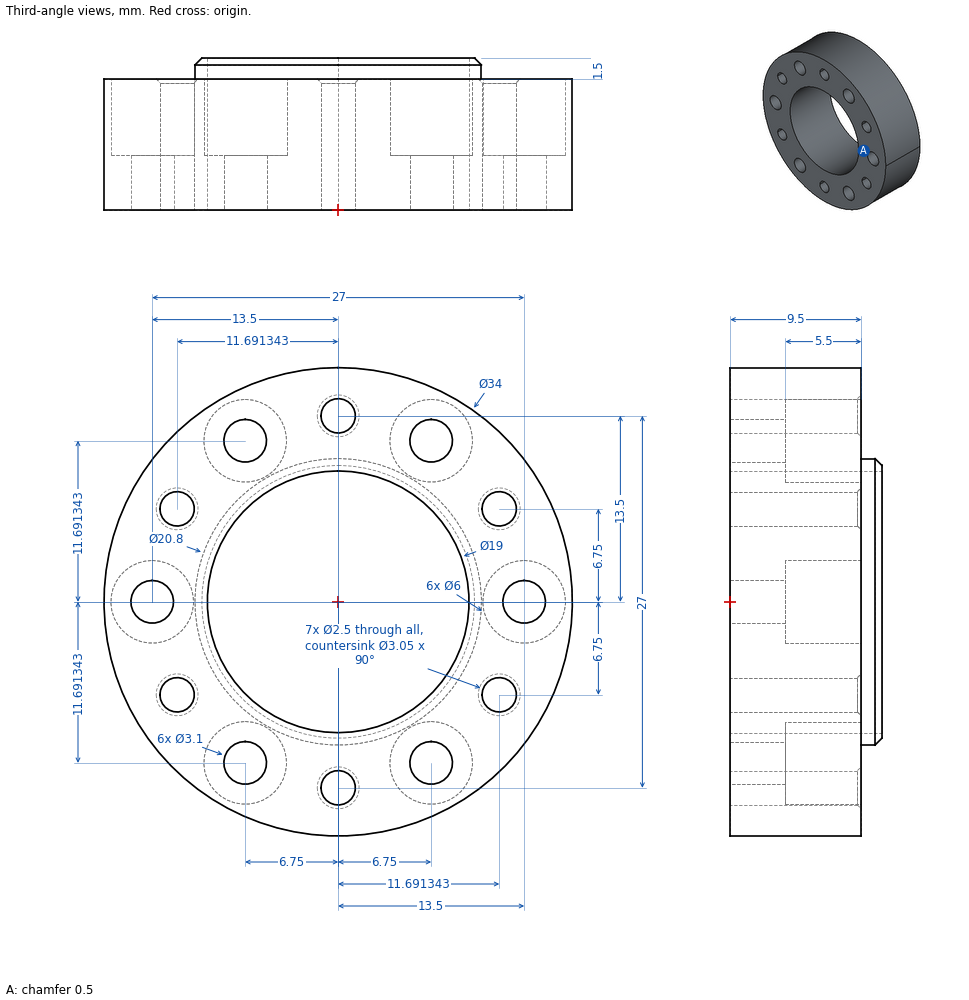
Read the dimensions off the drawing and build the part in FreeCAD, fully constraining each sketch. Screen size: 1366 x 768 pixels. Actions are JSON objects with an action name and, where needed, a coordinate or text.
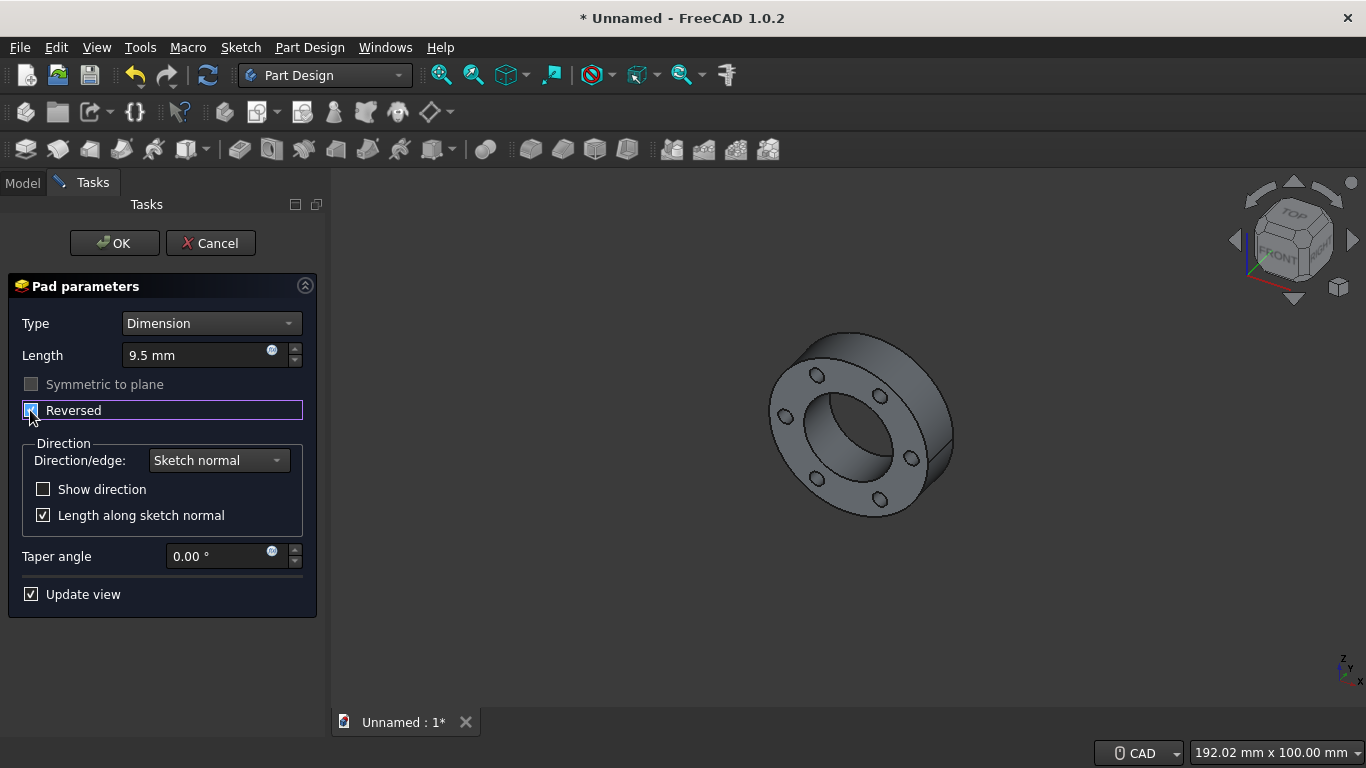
{"action": "left_click", "coordinate": [115, 243]}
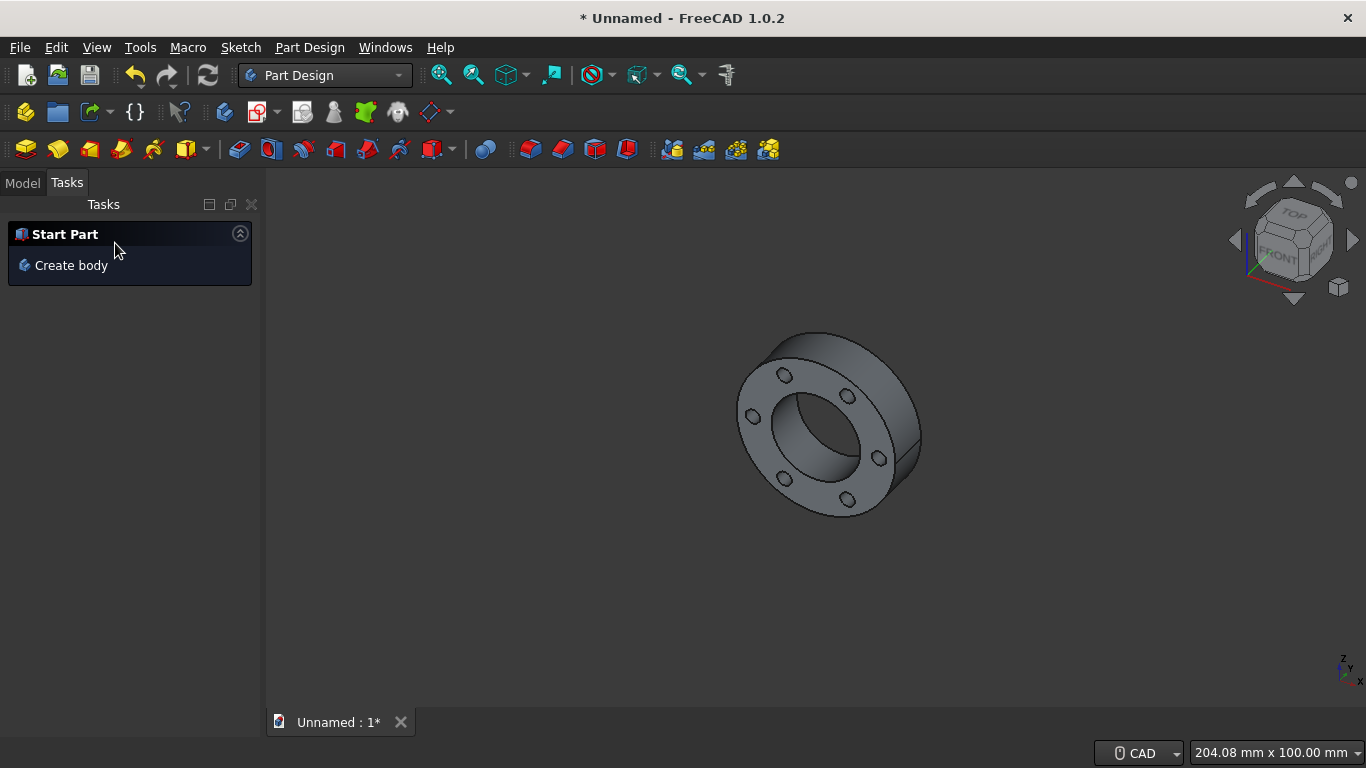
{"action": "left_click", "coordinate": [442, 76]}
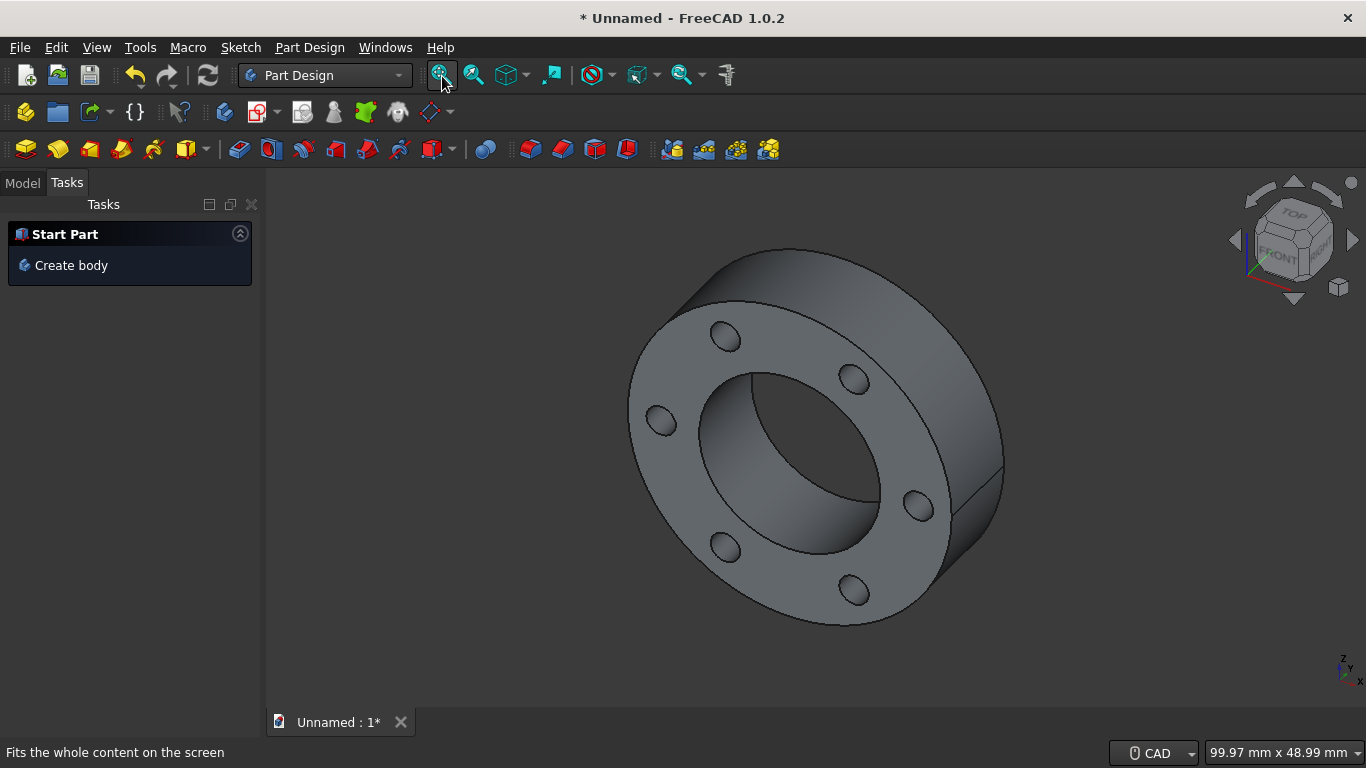
{"action": "key", "text": "4"}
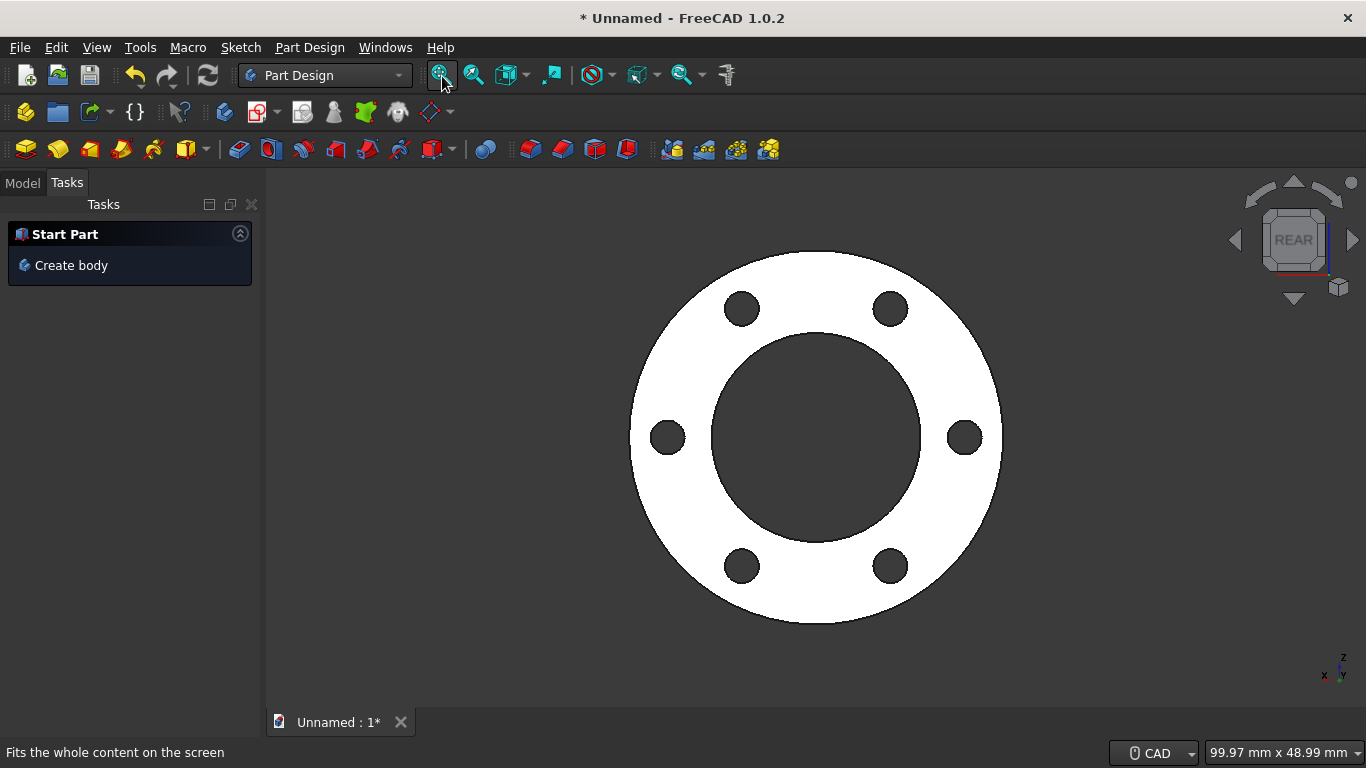
{"action": "left_click", "coordinate": [816, 597]}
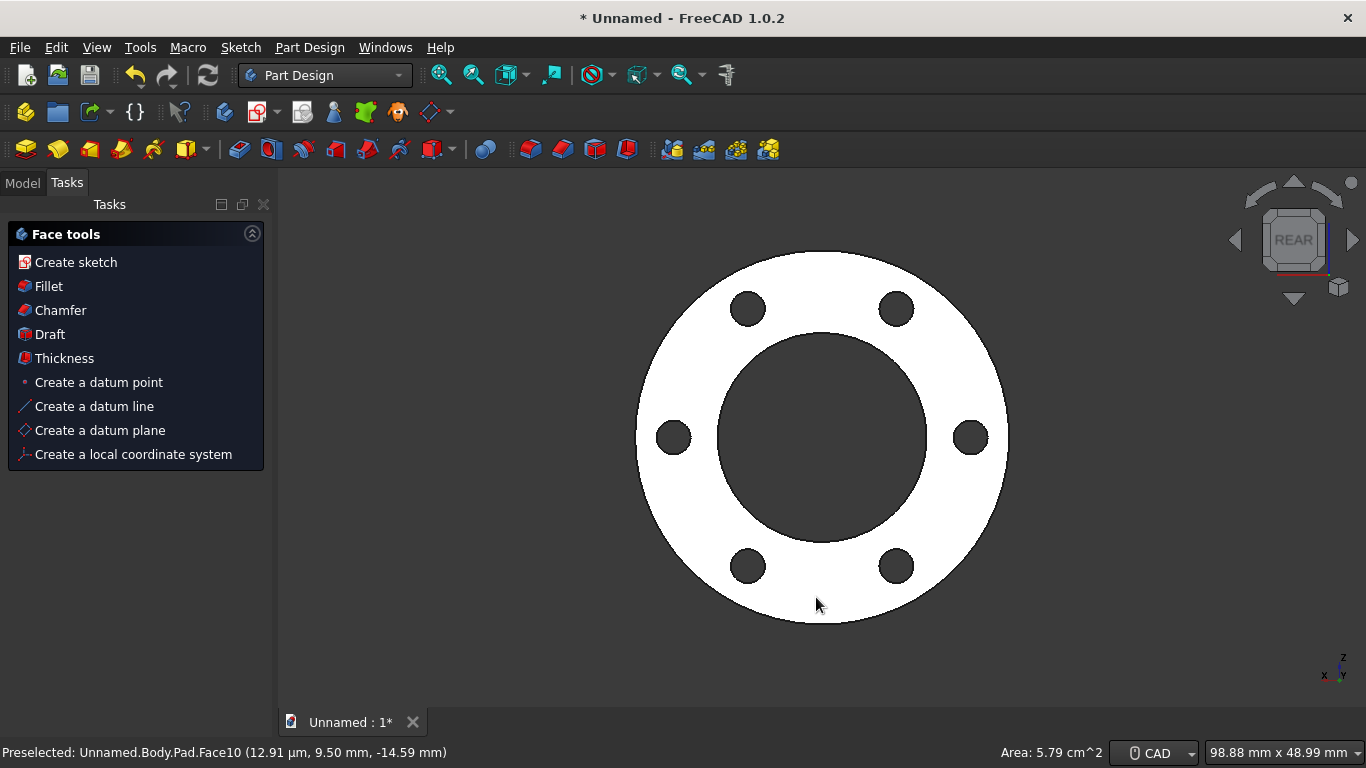
{"action": "left_click", "coordinate": [258, 112]}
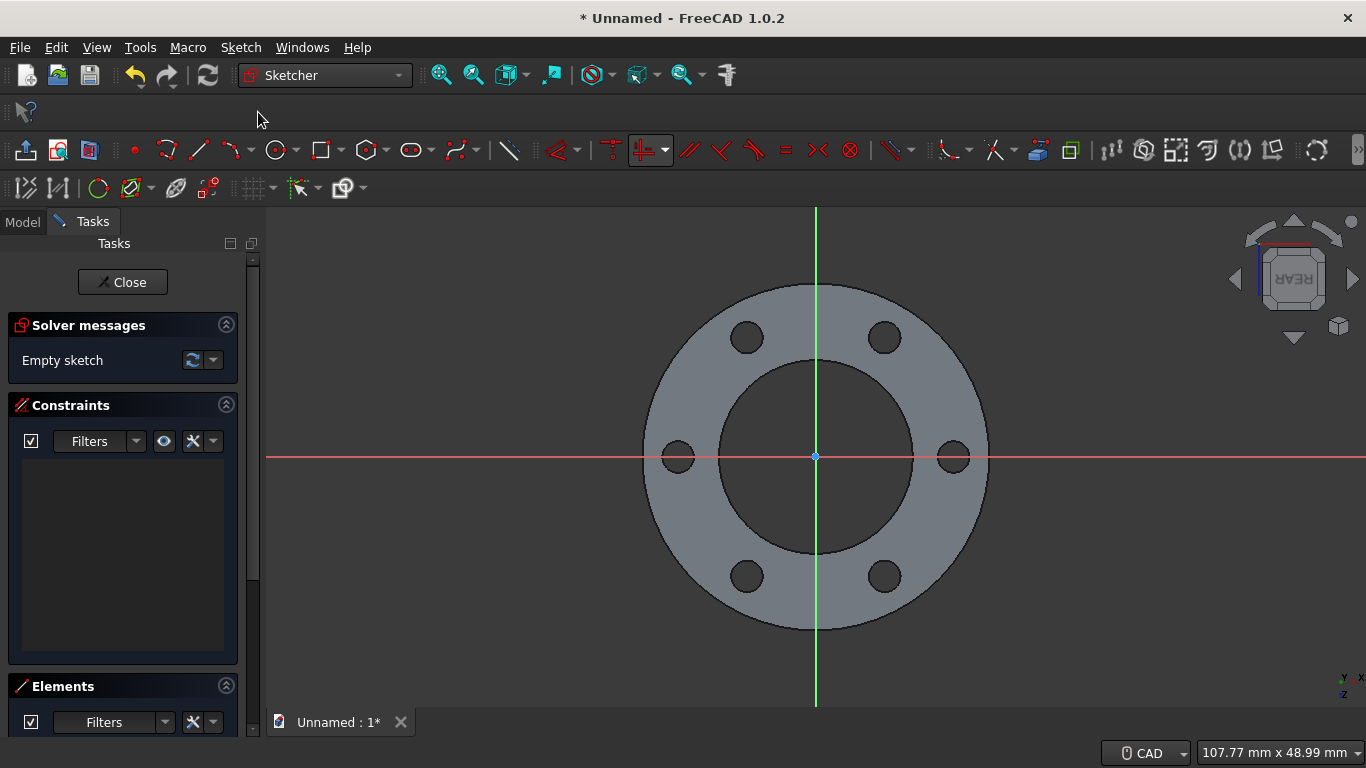
{"action": "left_click", "coordinate": [276, 150]}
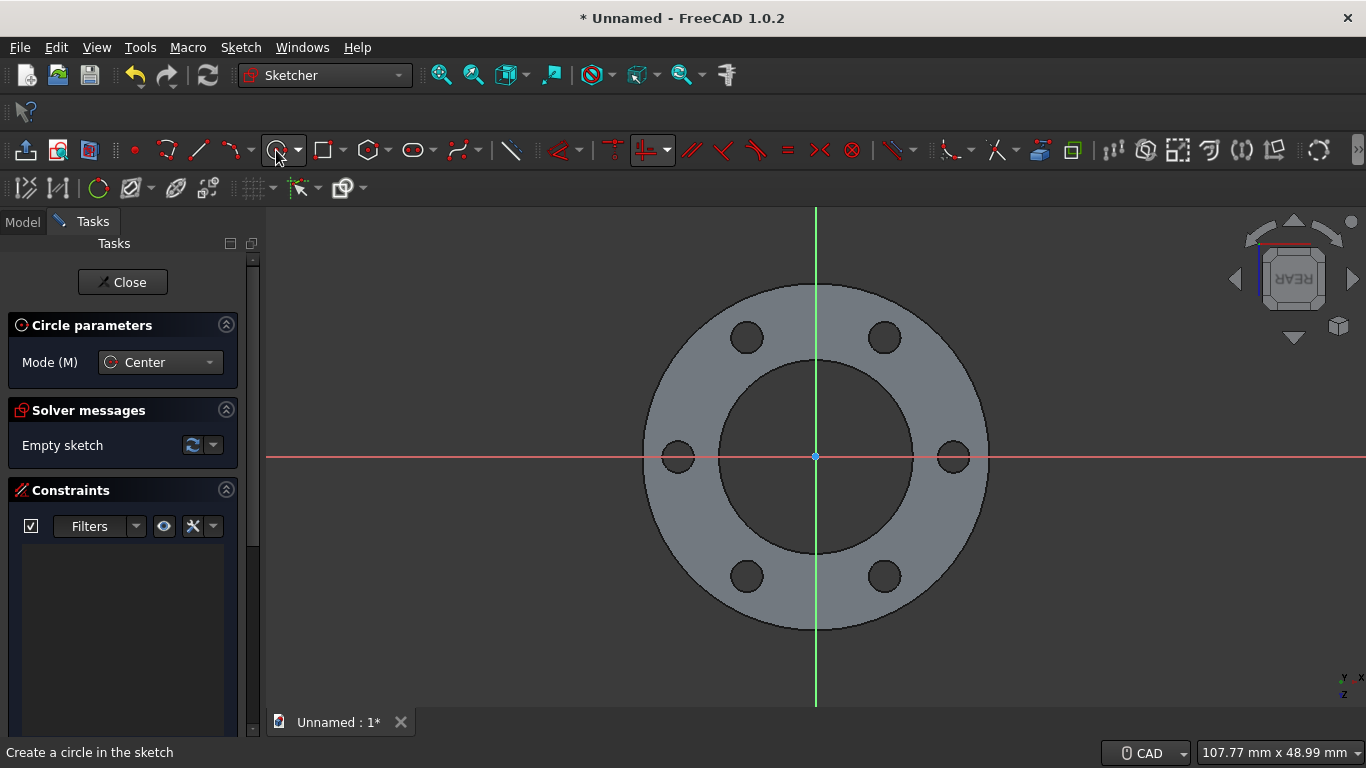
{"action": "scroll", "coordinate": [935, 388], "scroll_direction": "up", "scroll_amount": 3}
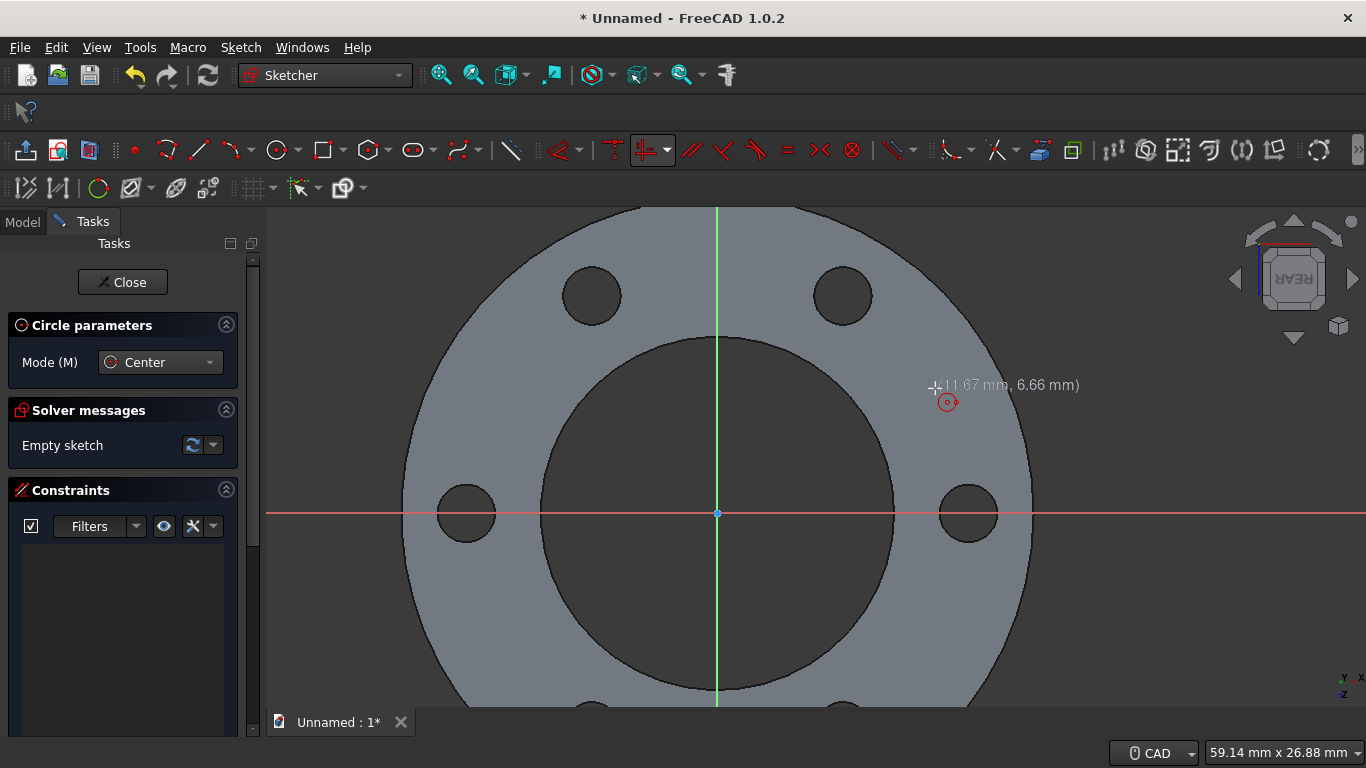
{"action": "left_click", "coordinate": [935, 388]}
{"action": "mouse_move", "coordinate": [951, 371]}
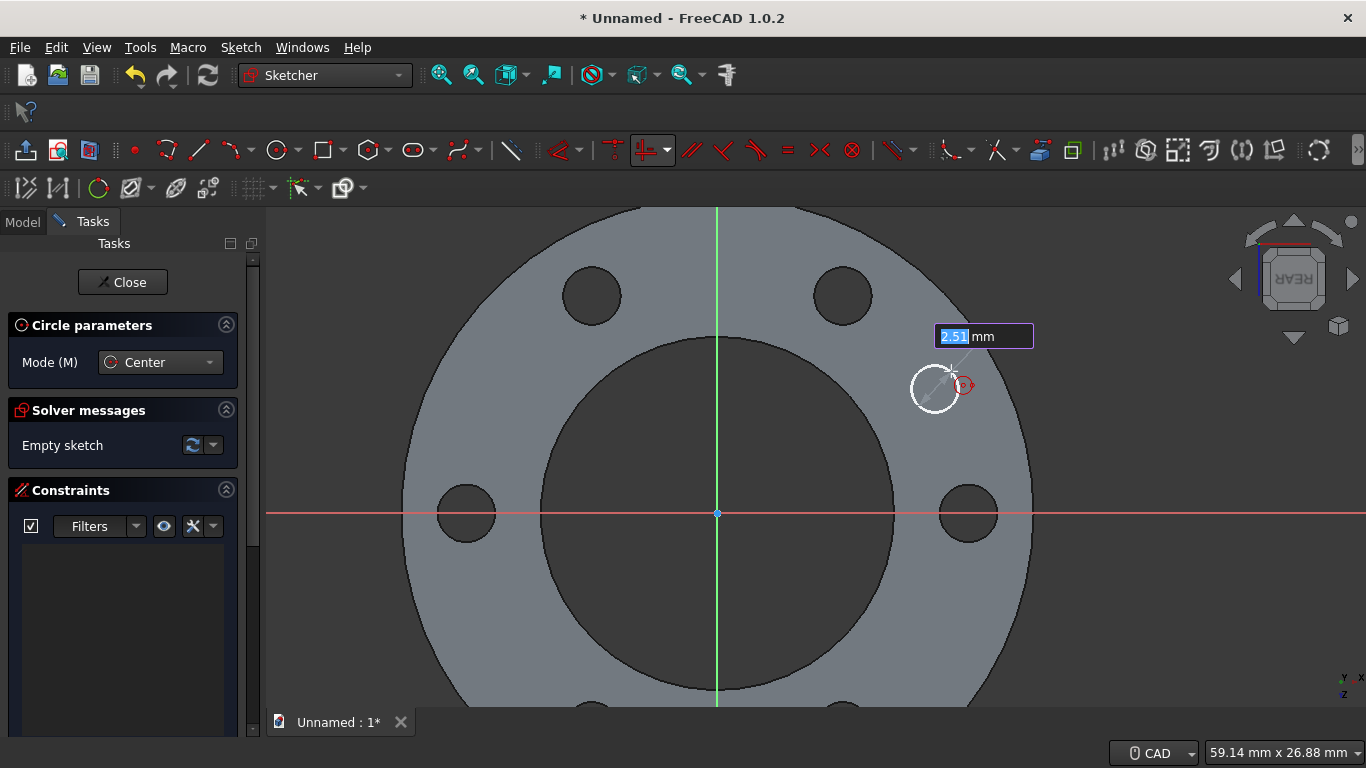
{"action": "type", "text": "2.5"}
{"action": "key", "text": "Return"}